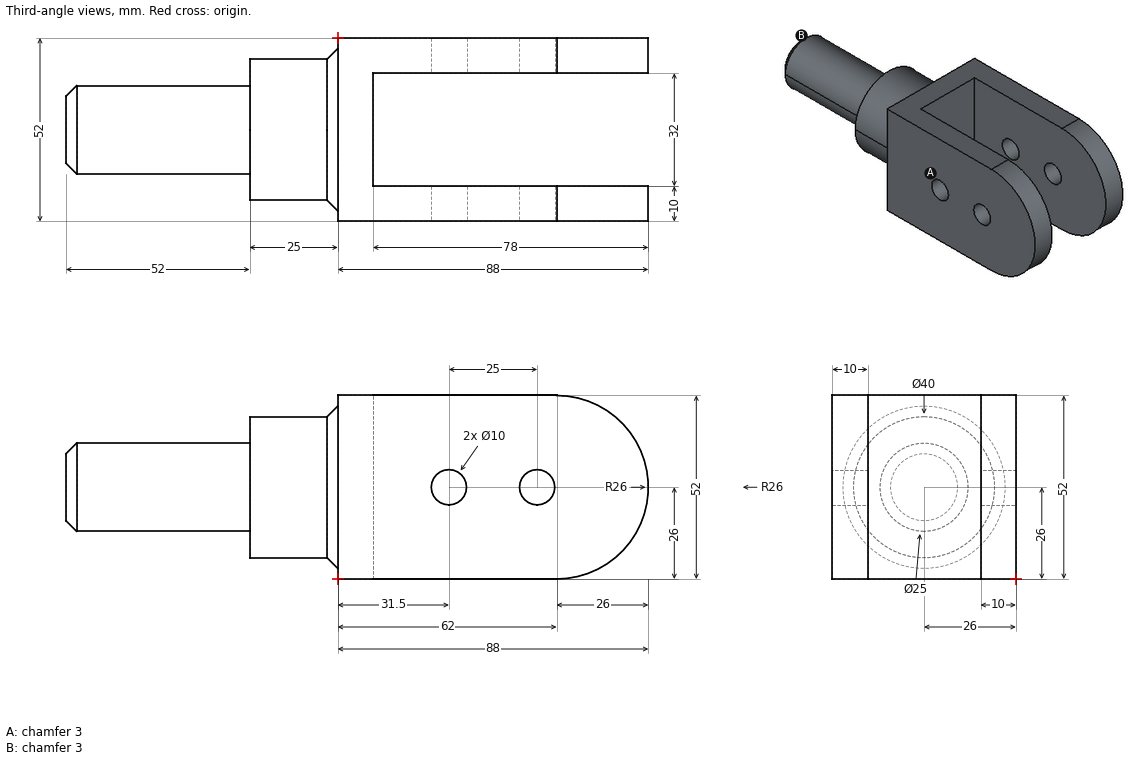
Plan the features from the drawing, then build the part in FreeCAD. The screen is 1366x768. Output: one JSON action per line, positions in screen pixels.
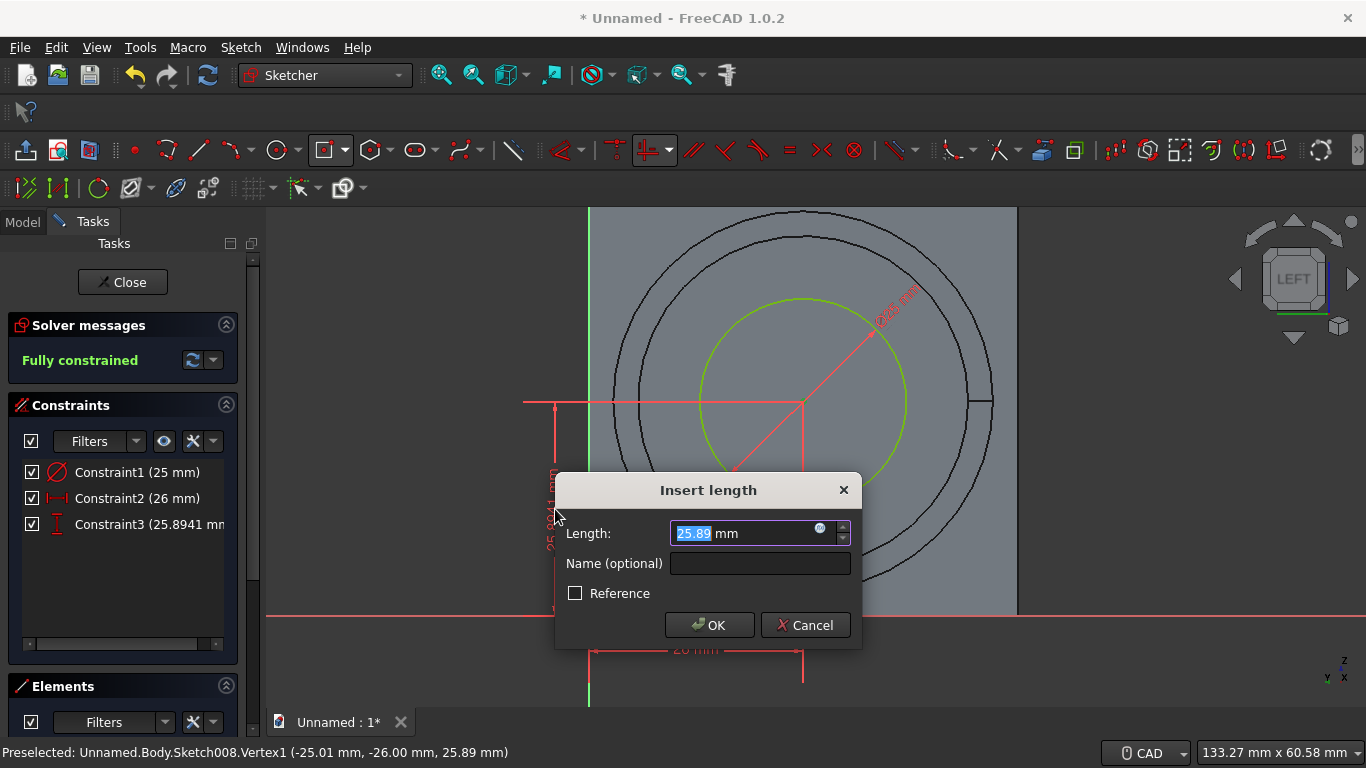
{"action": "type", "text": "26"}
{"action": "key", "text": "Return"}
{"action": "key", "text": "Escape"}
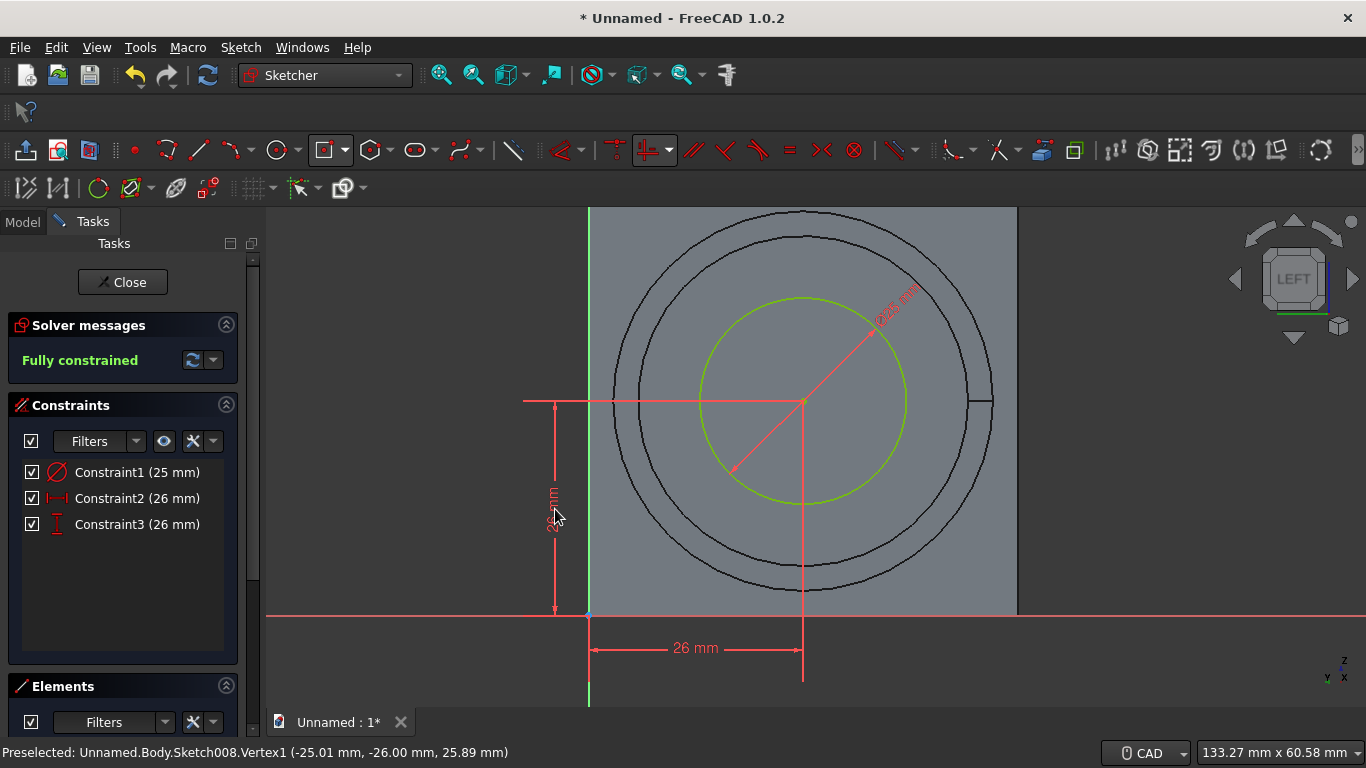
{"action": "left_click", "coordinate": [123, 282]}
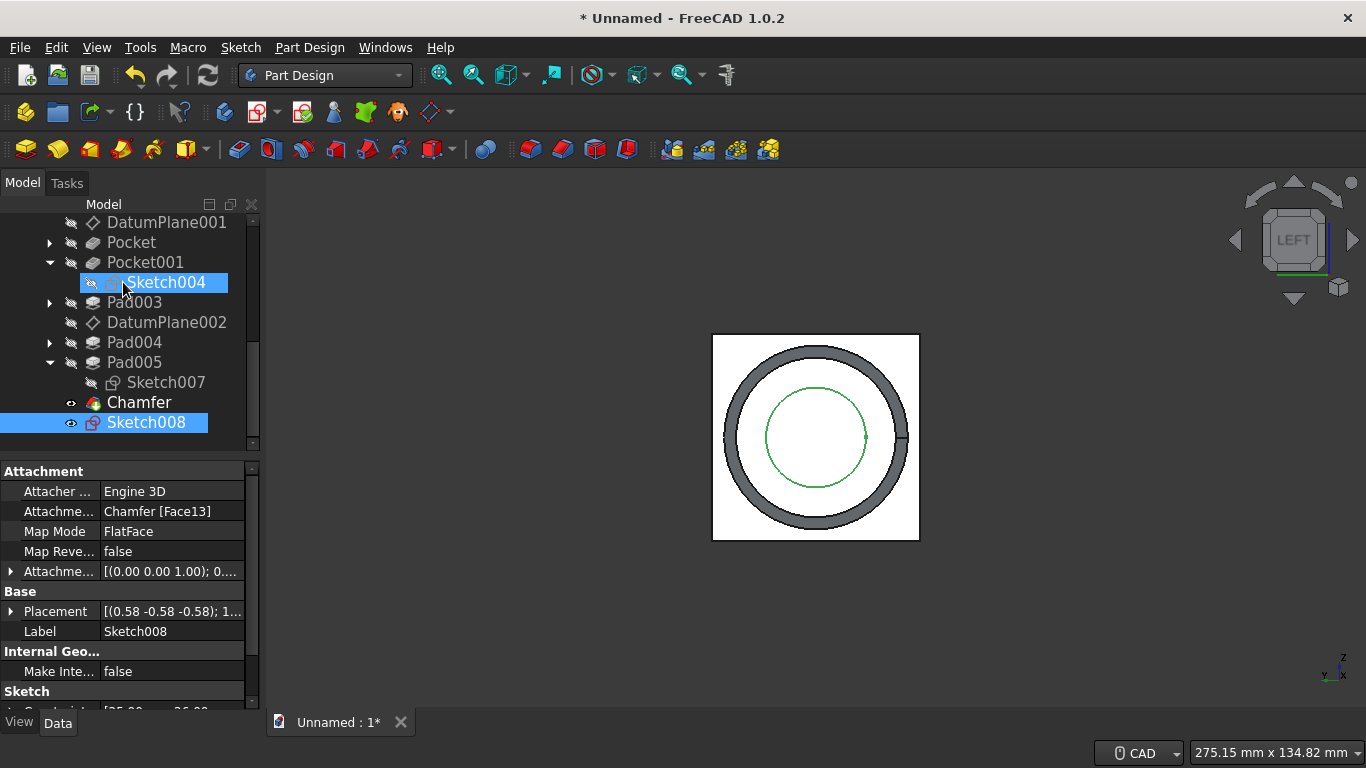
{"action": "left_click", "coordinate": [26, 150]}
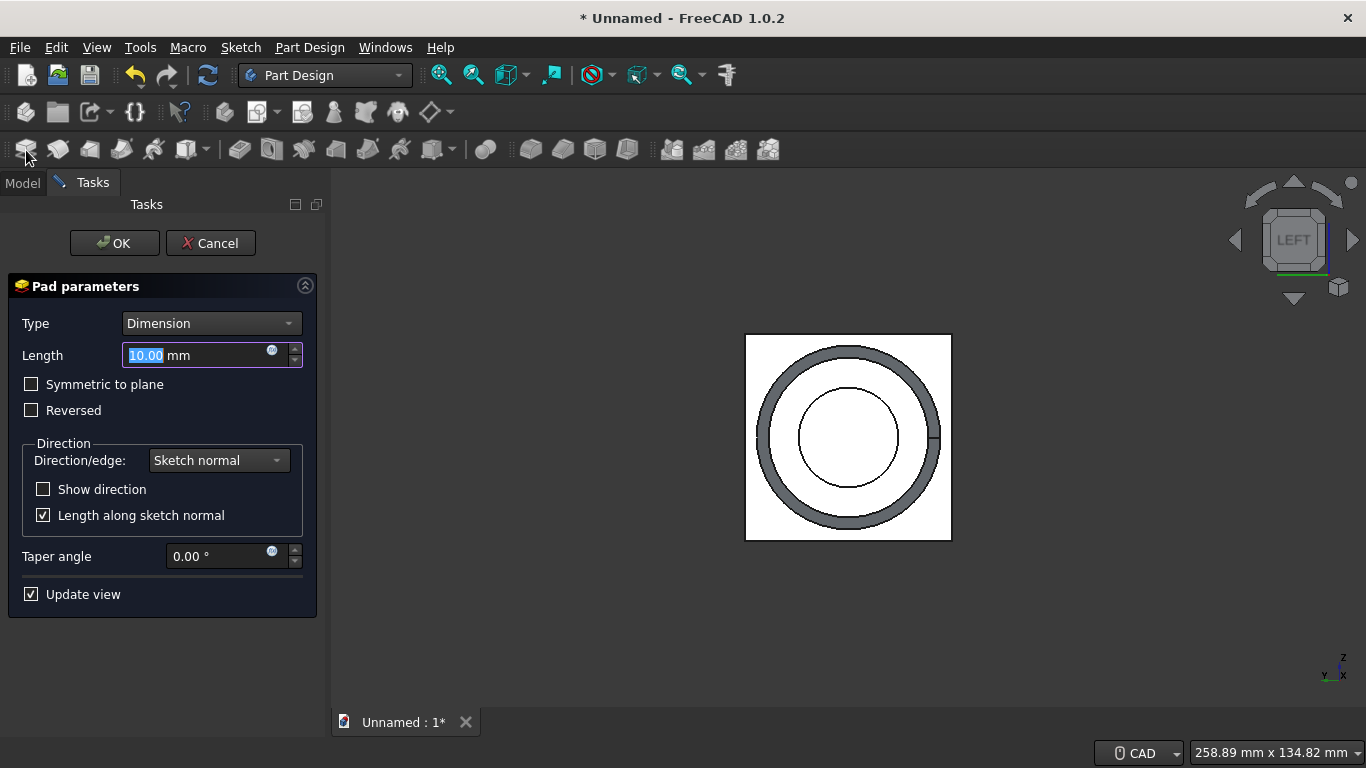
{"action": "type", "text": "52"}
{"action": "key", "text": "Tab"}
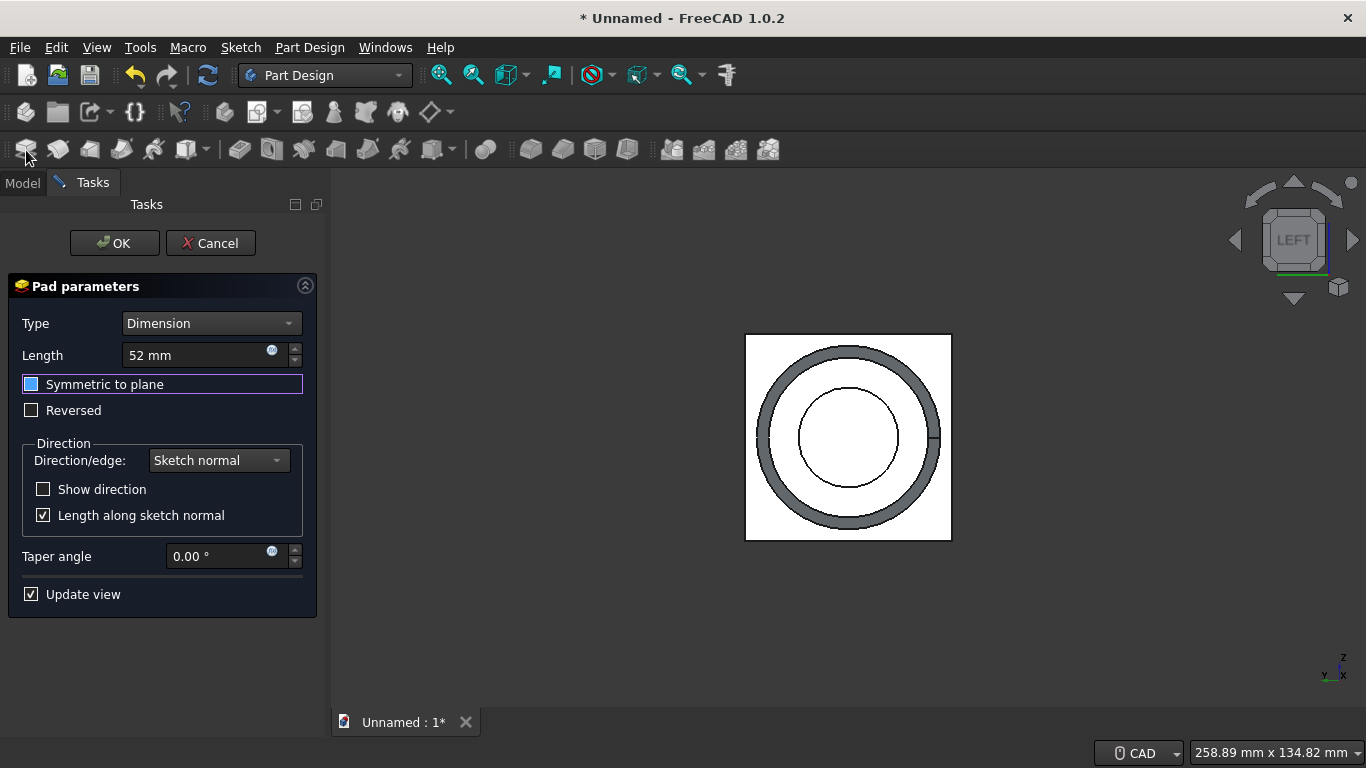
{"action": "left_click", "coordinate": [115, 243]}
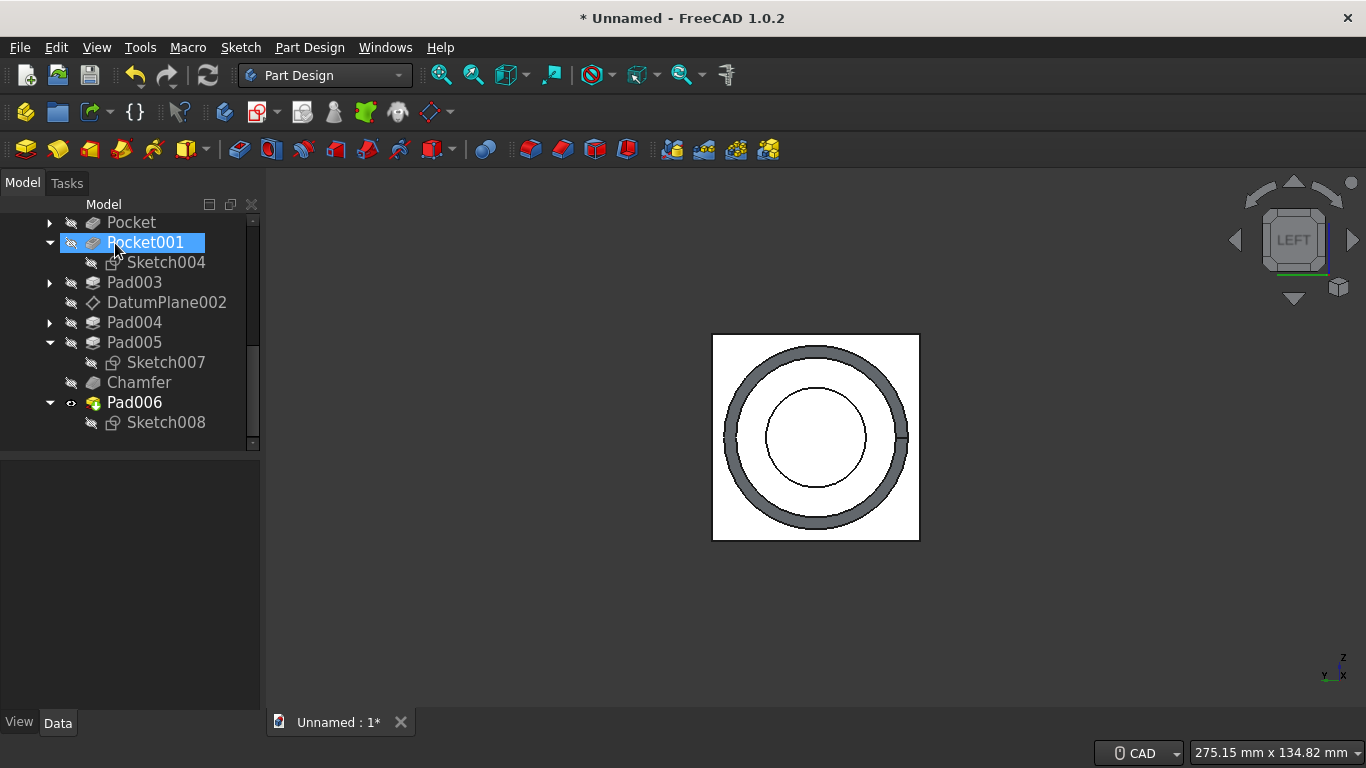
{"action": "left_click", "coordinate": [442, 76]}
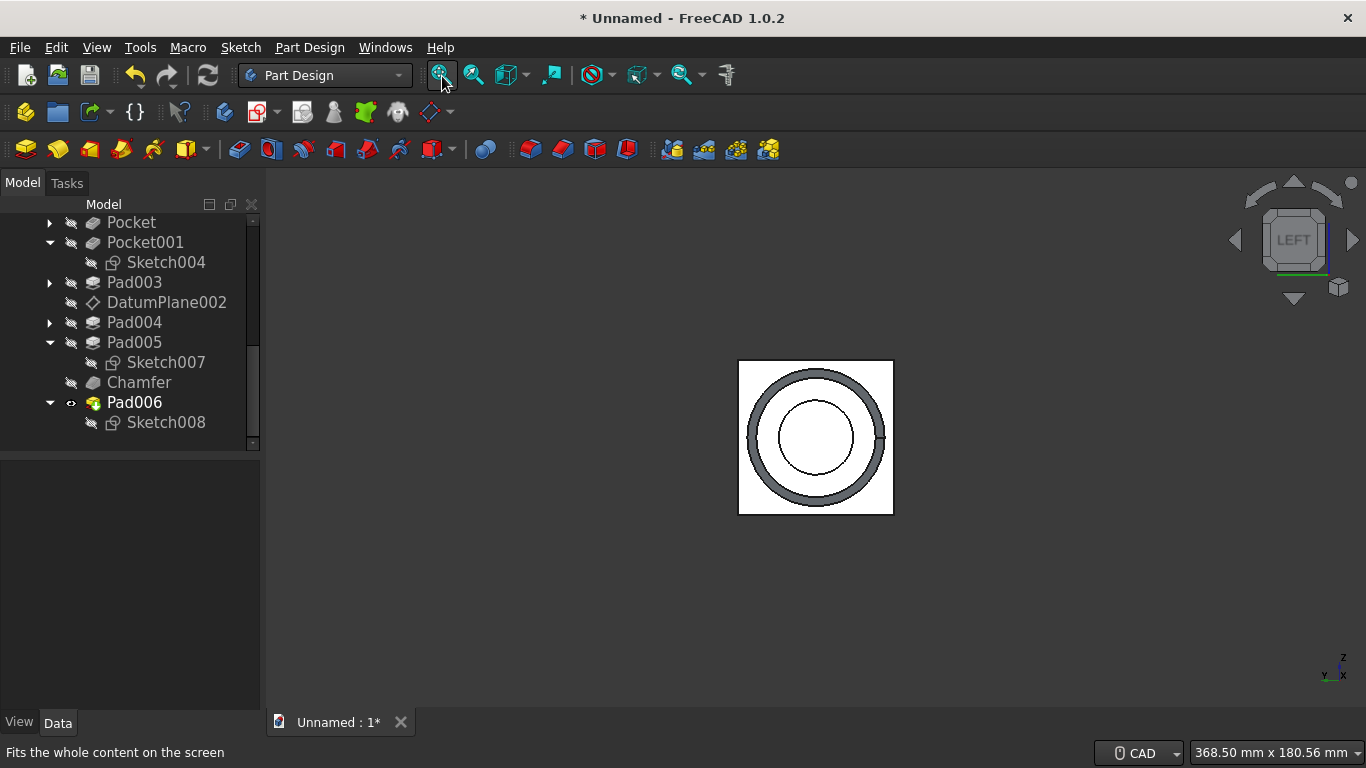
{"action": "left_click", "coordinate": [779, 436]}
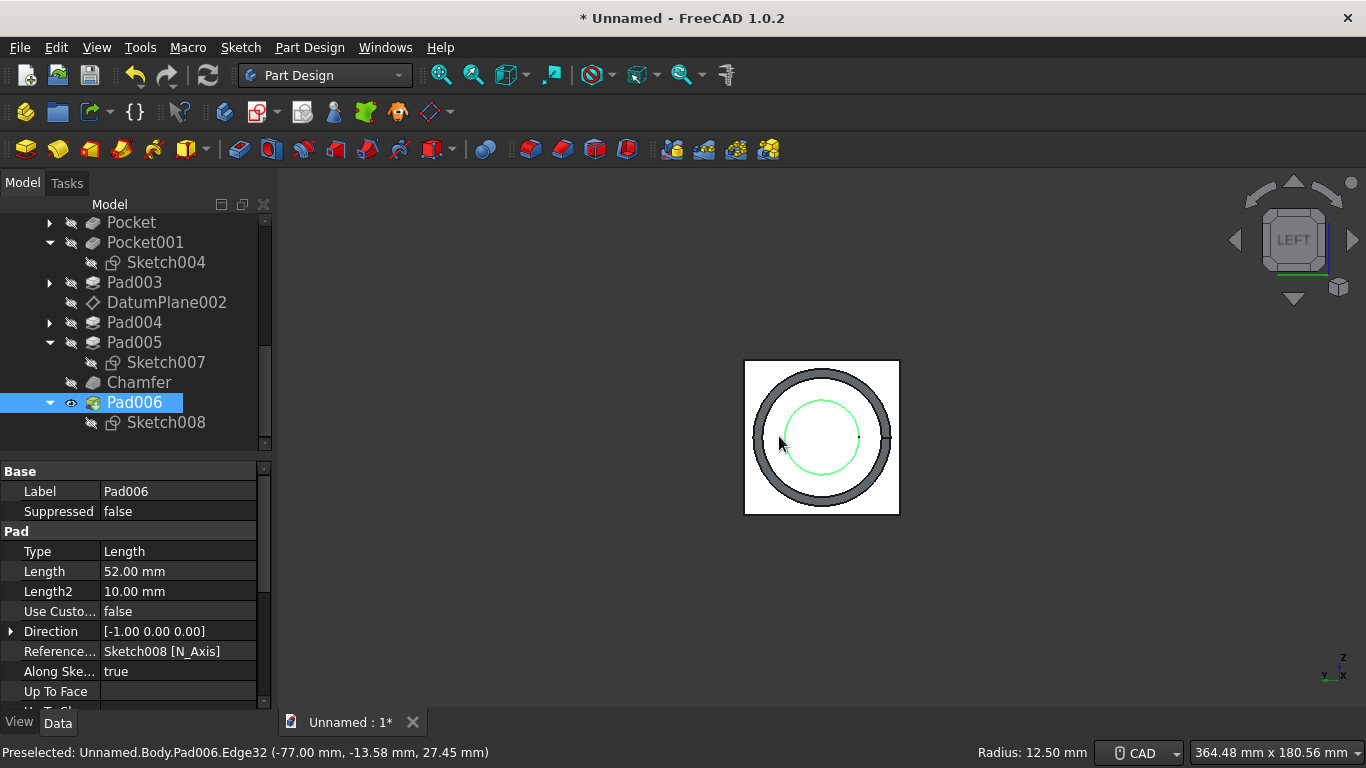
{"action": "left_click", "coordinate": [564, 150]}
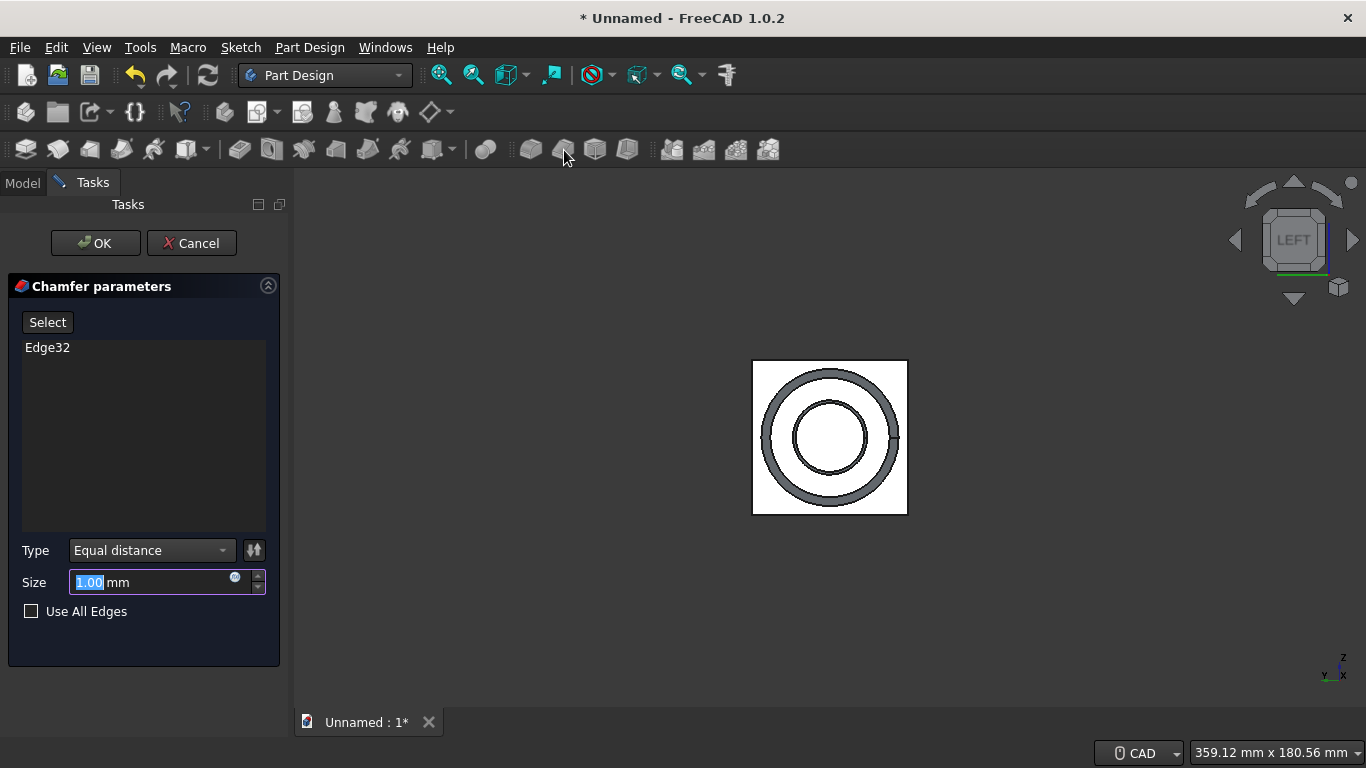
{"action": "type", "text": "3"}
{"action": "key", "text": "Tab"}